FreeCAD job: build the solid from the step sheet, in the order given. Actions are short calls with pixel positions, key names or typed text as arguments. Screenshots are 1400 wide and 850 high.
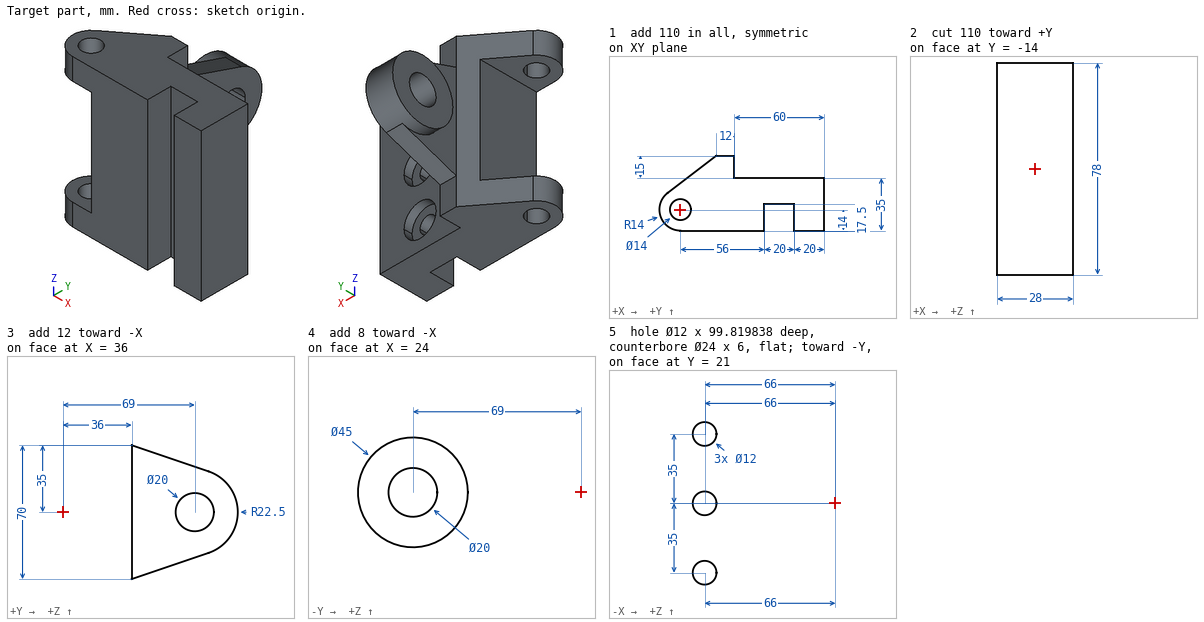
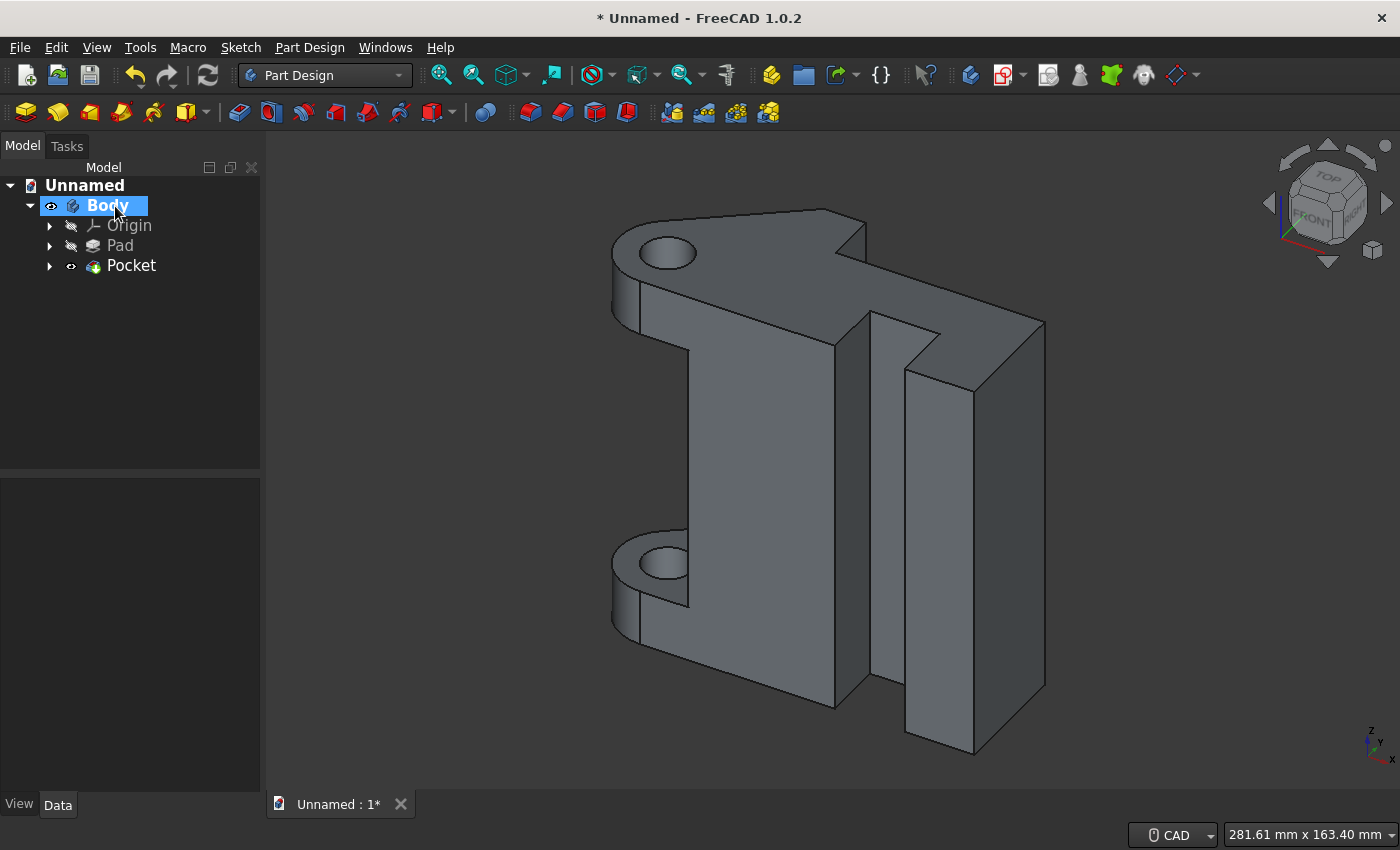
key(0)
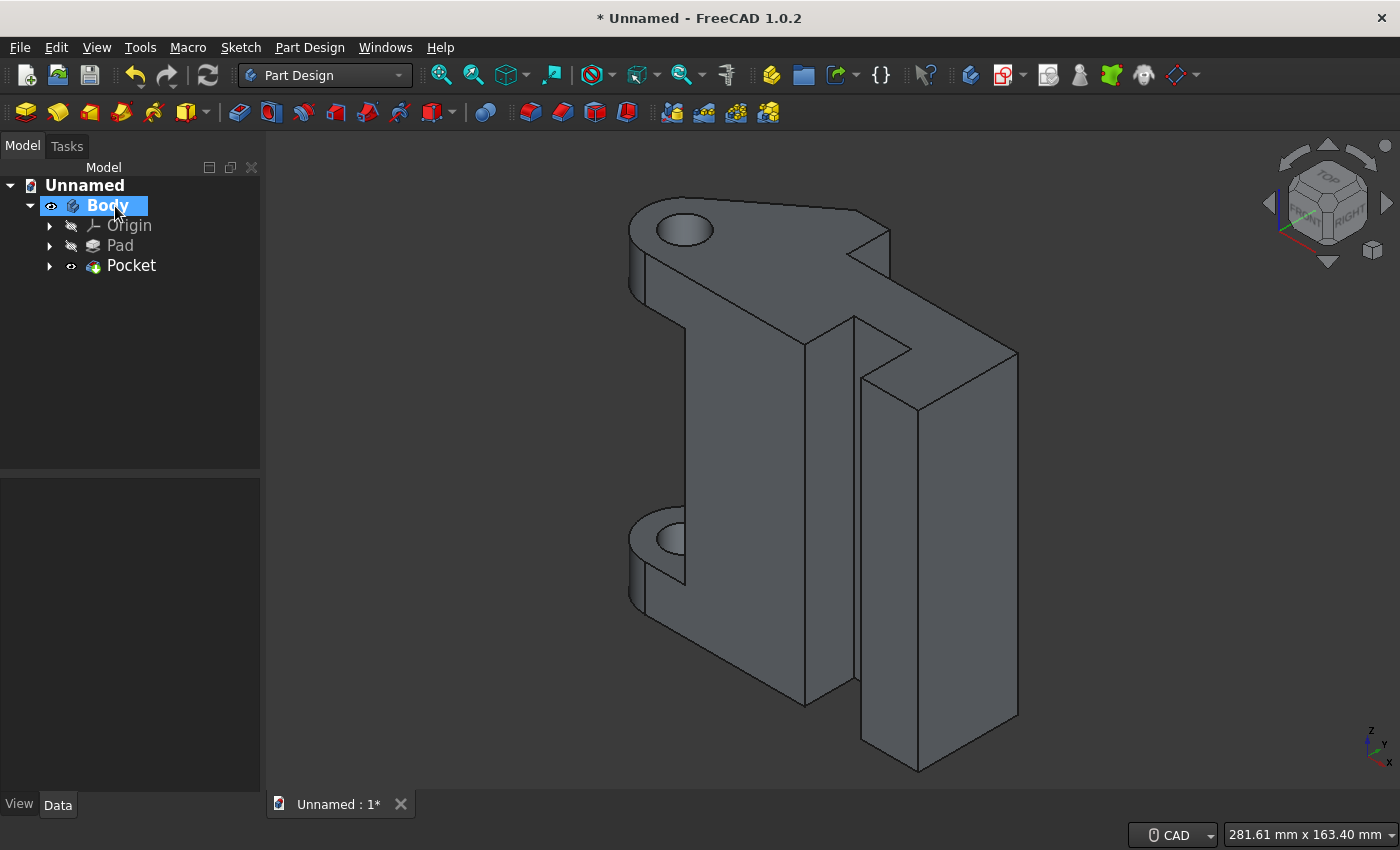
key(3)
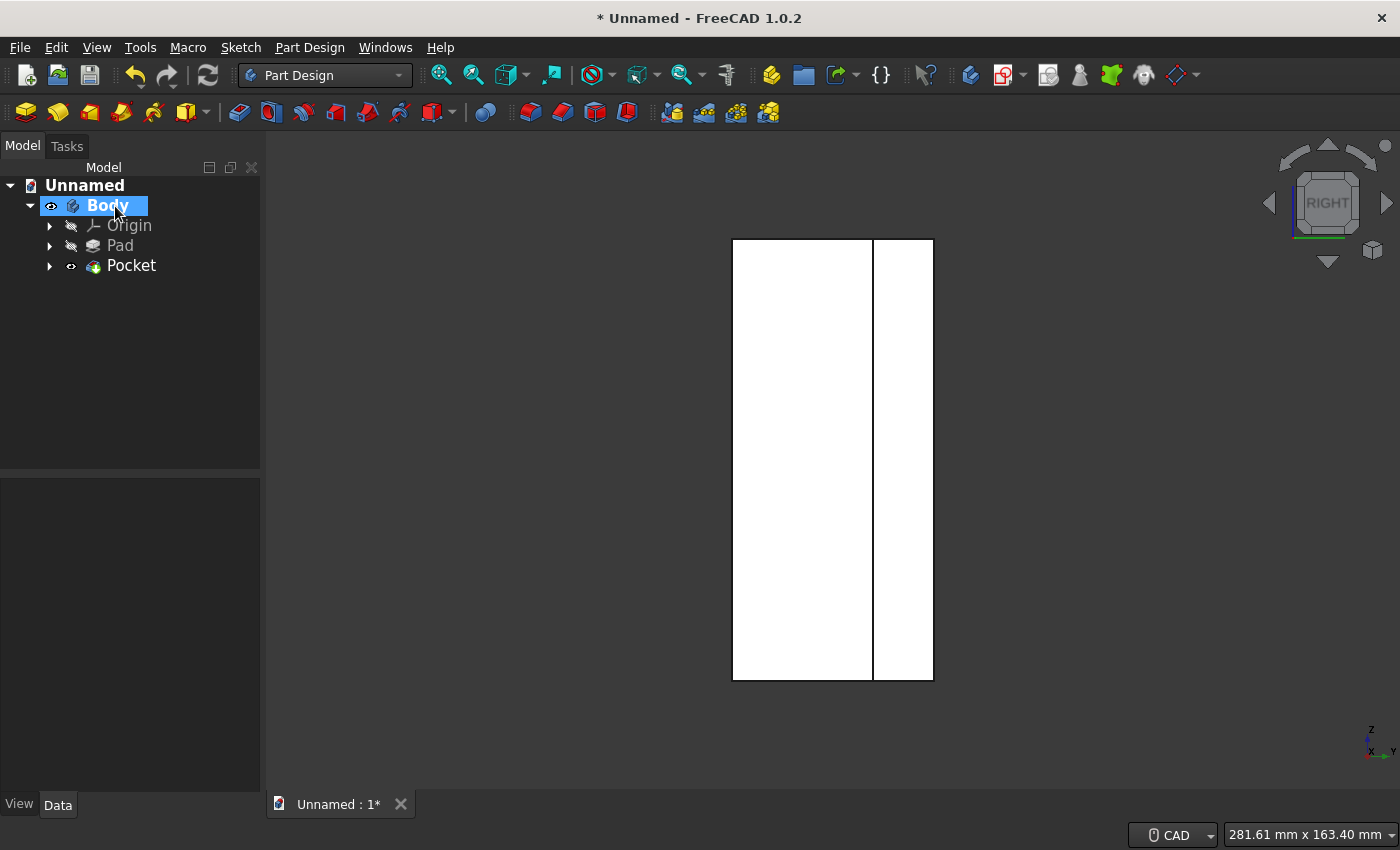
click(903, 269)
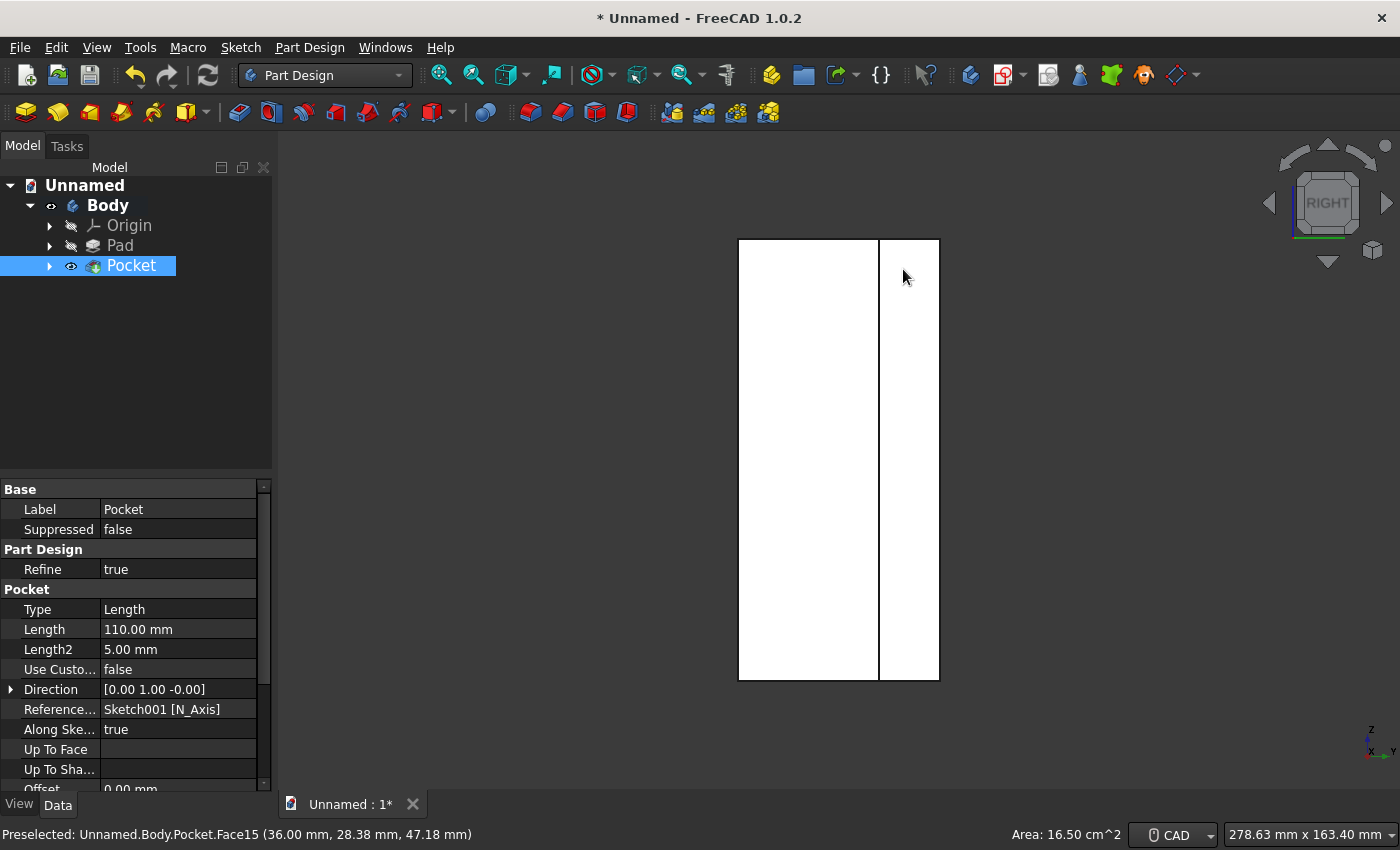
click(1004, 76)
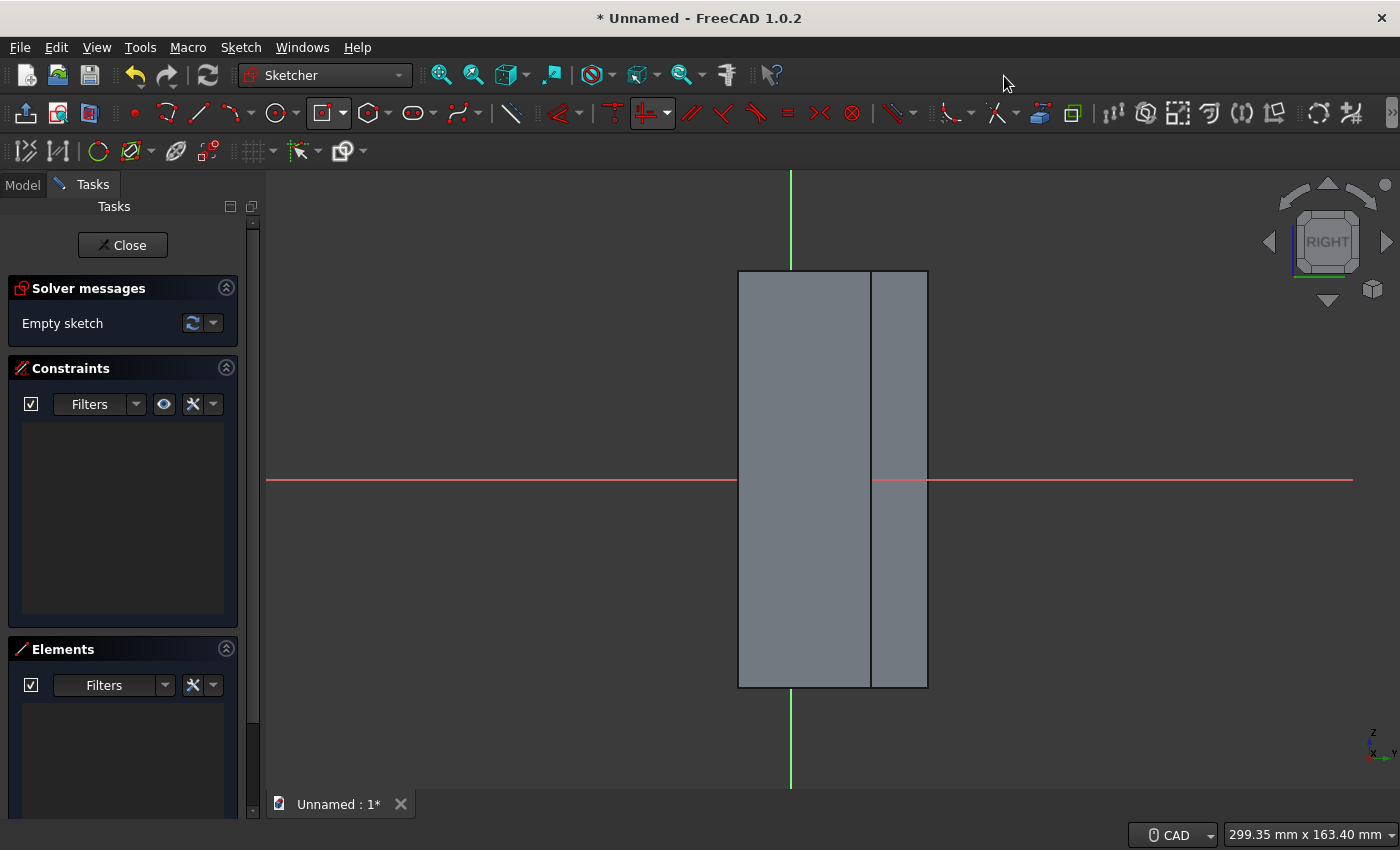
scroll(1235, 480, up, 2)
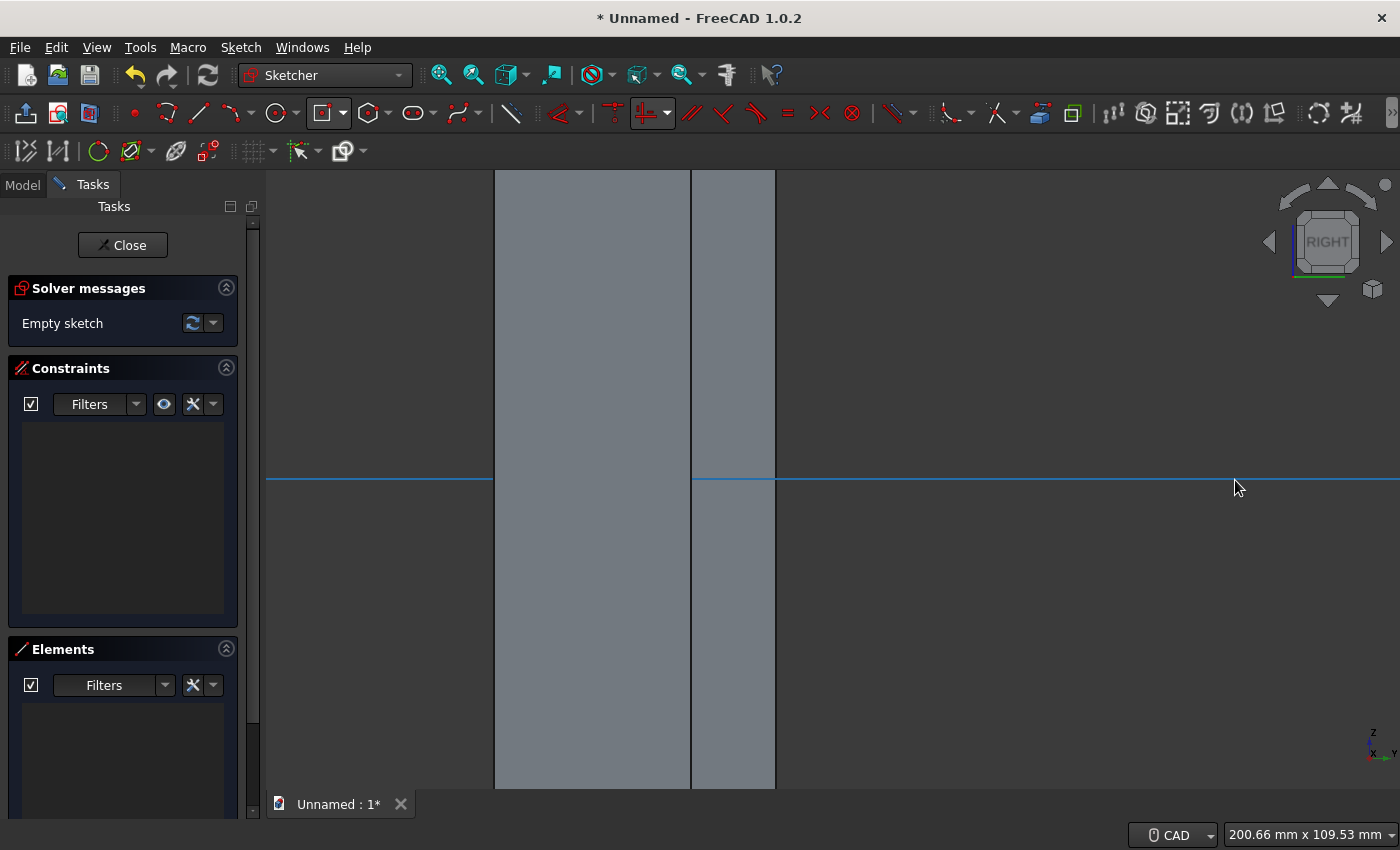
click(168, 114)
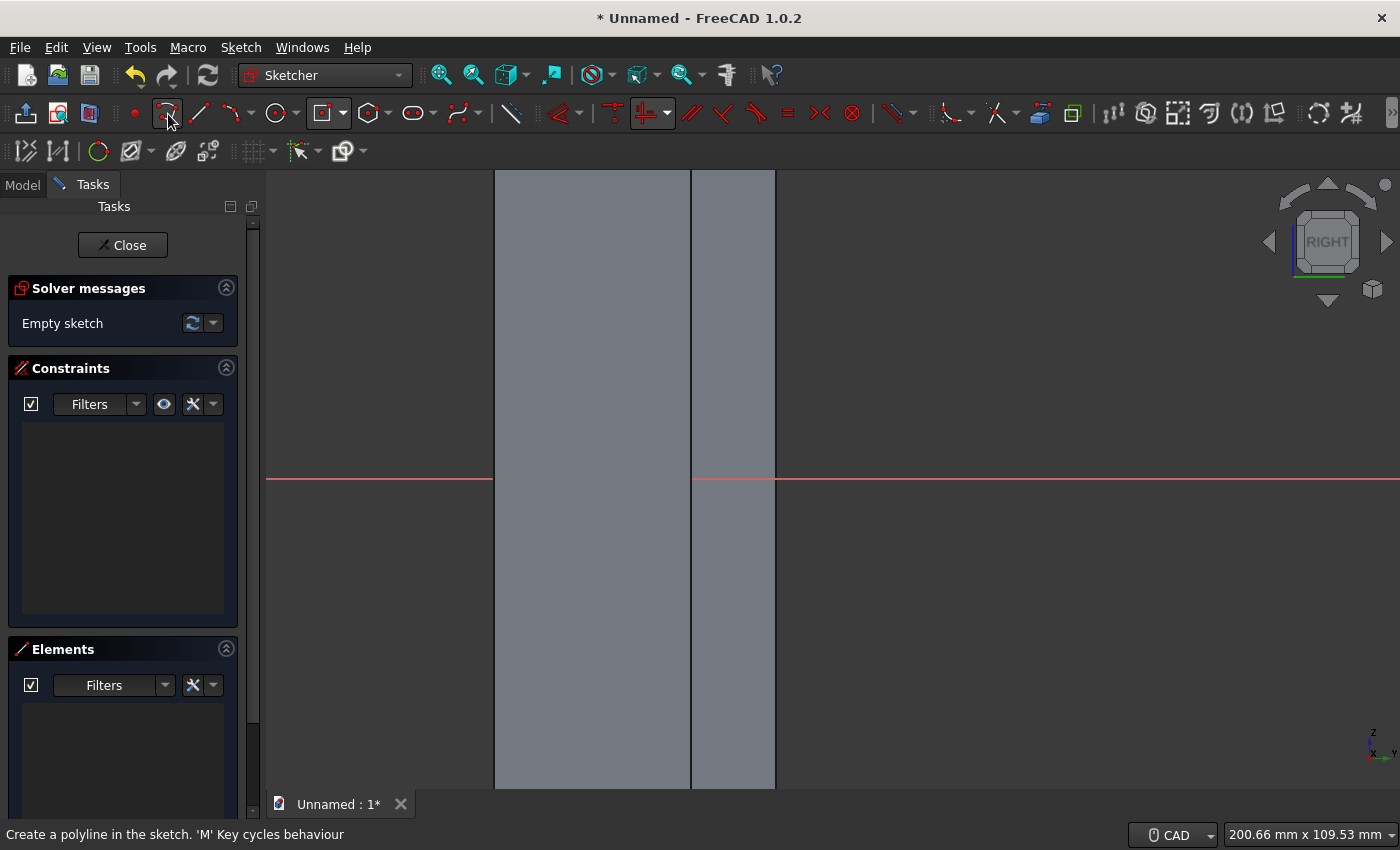
click(1004, 359)
click(776, 281)
click(776, 677)
click(1004, 599)
right_click(1004, 599)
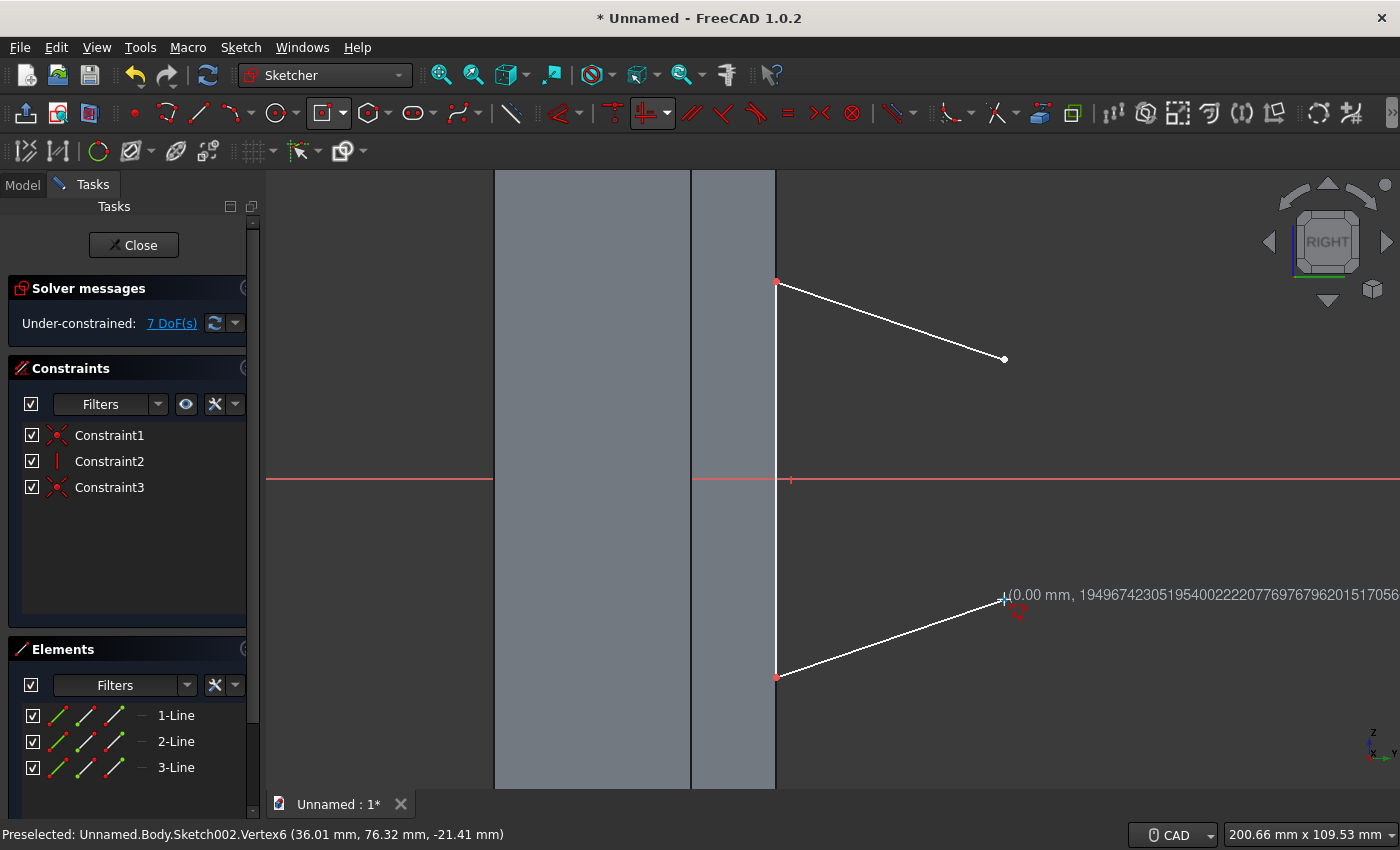
click(232, 114)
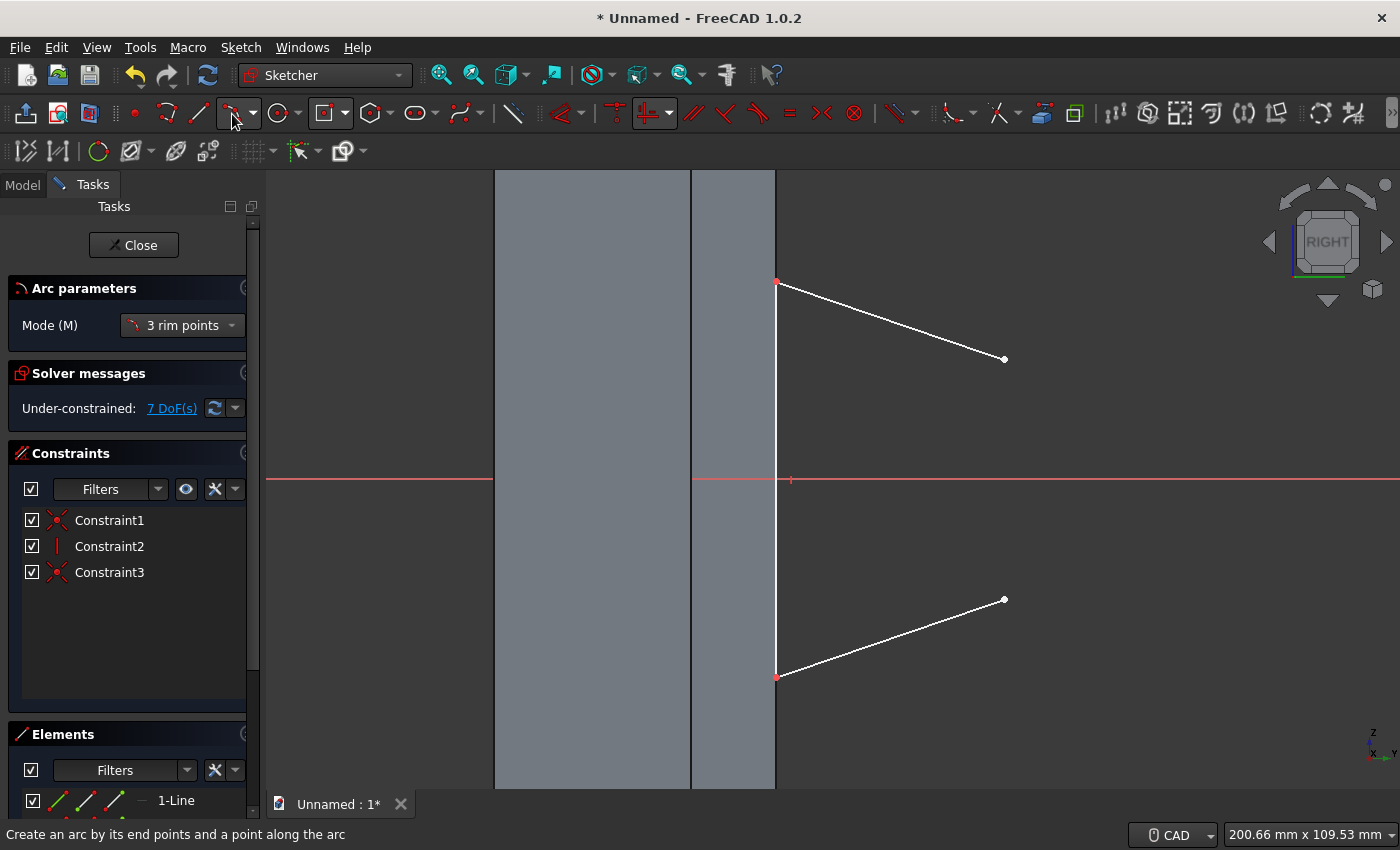
click(1004, 600)
click(1004, 360)
click(1086, 510)